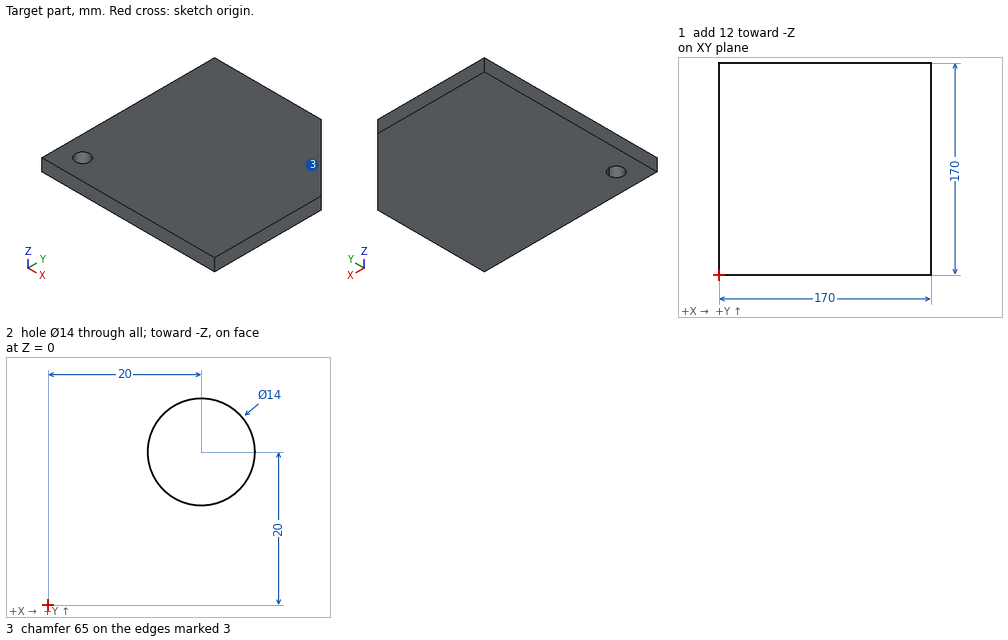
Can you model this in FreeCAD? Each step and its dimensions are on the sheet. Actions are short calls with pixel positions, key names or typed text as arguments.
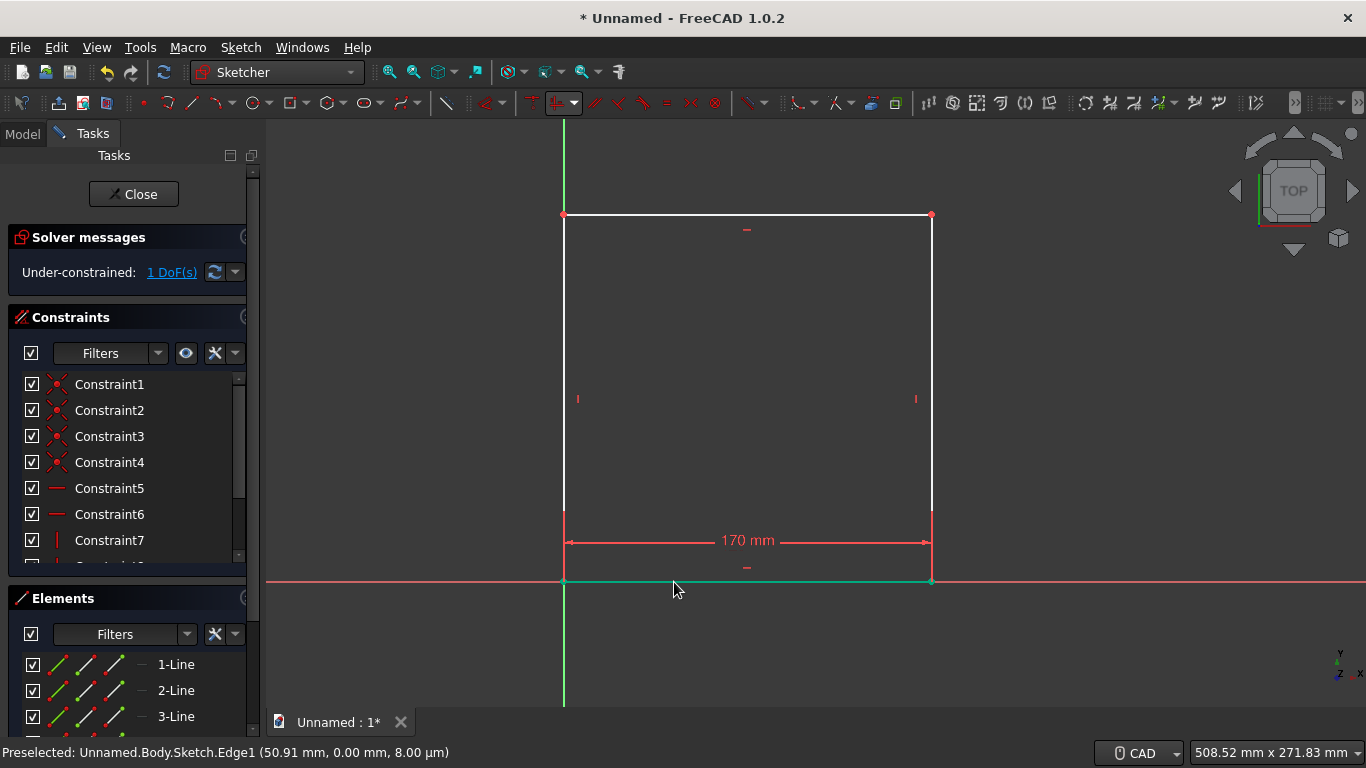
click(932, 472)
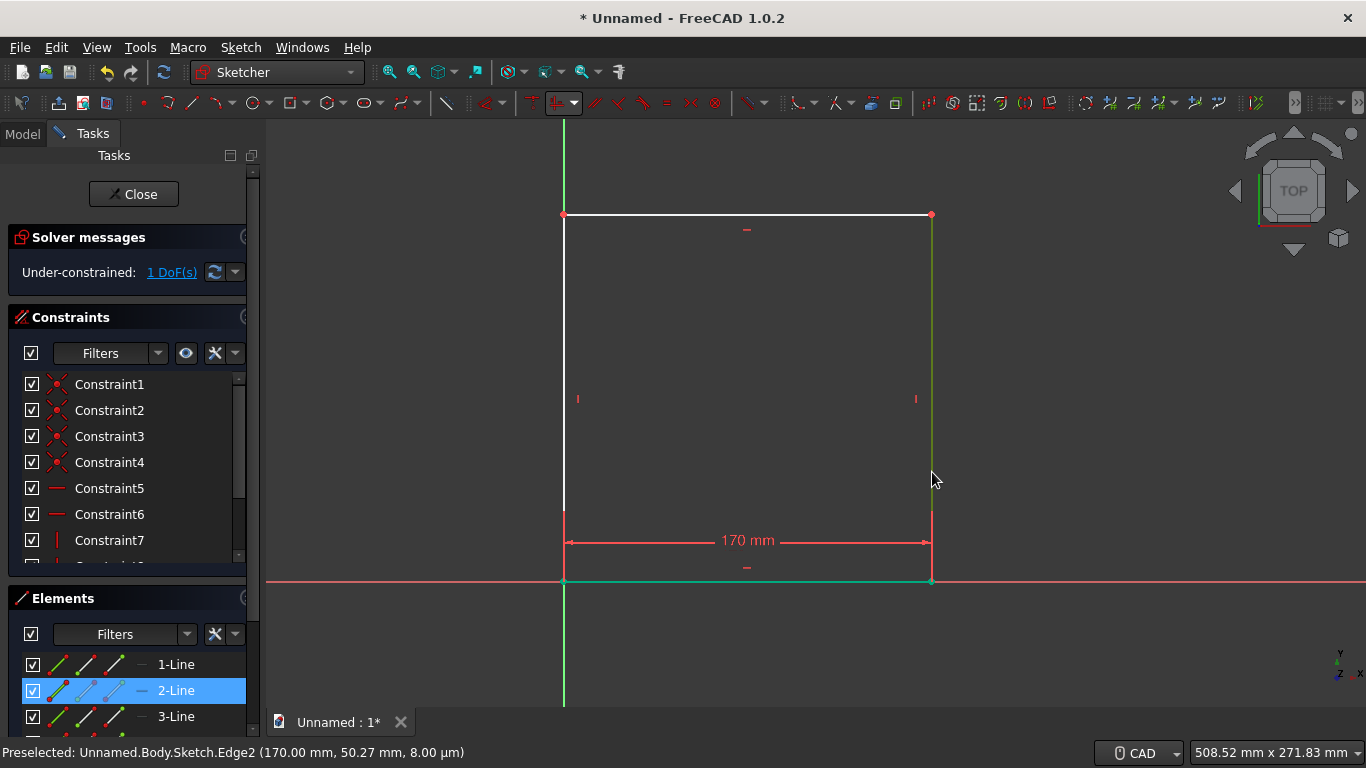
key(i)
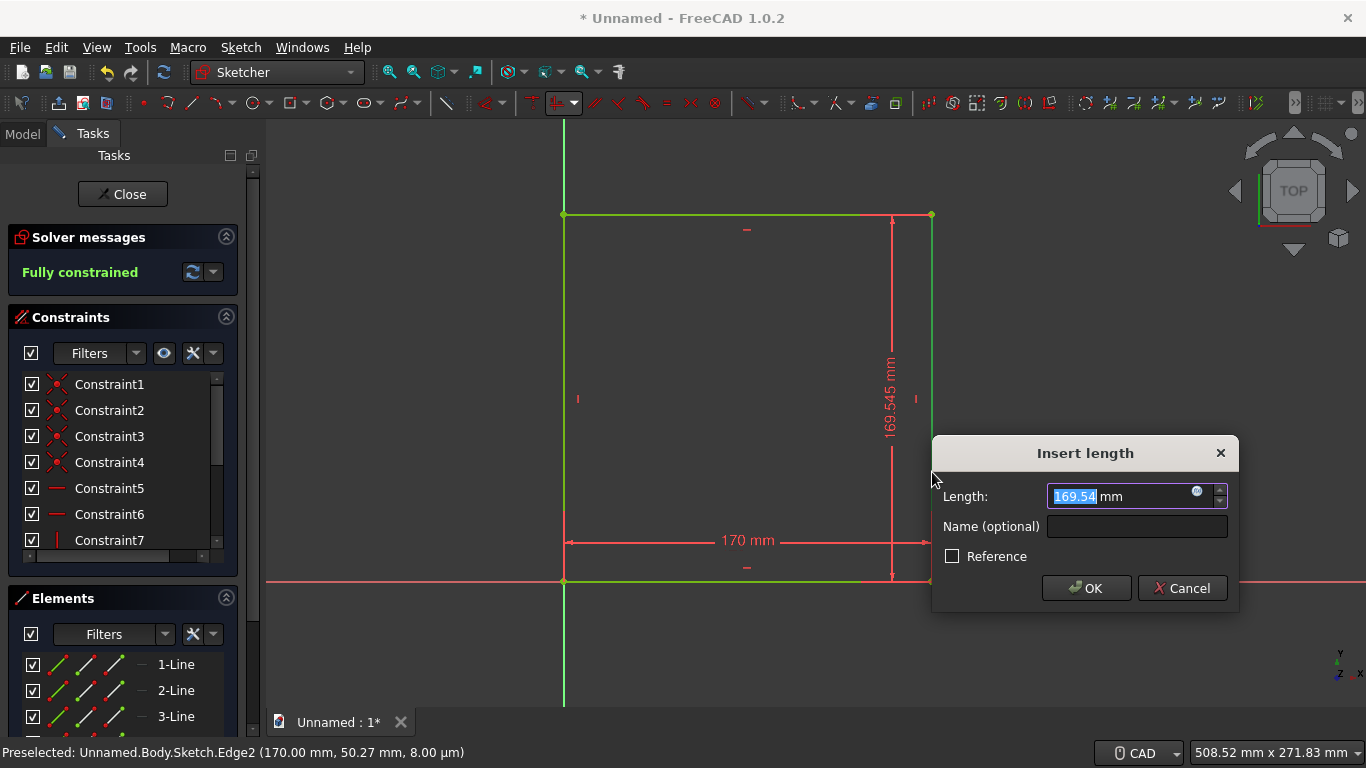
text(170)
key(Return)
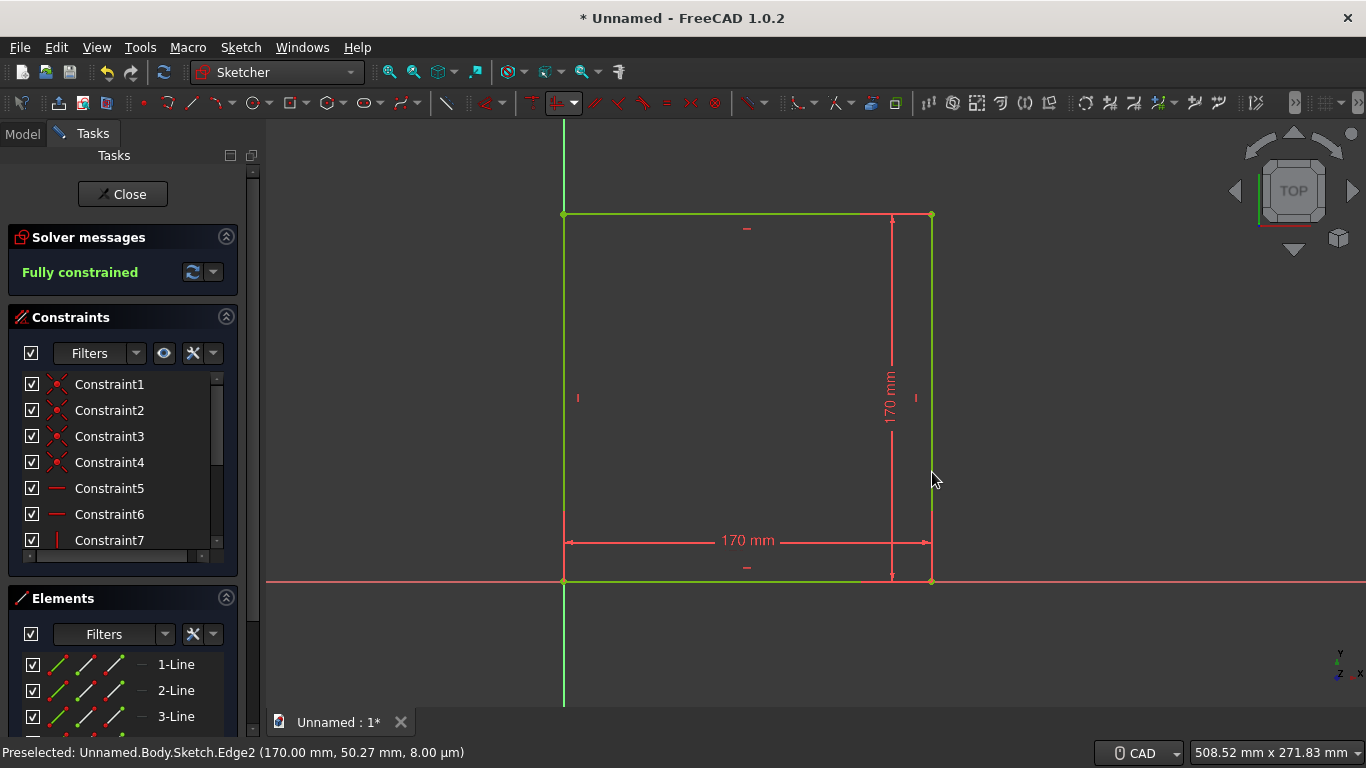
click(123, 194)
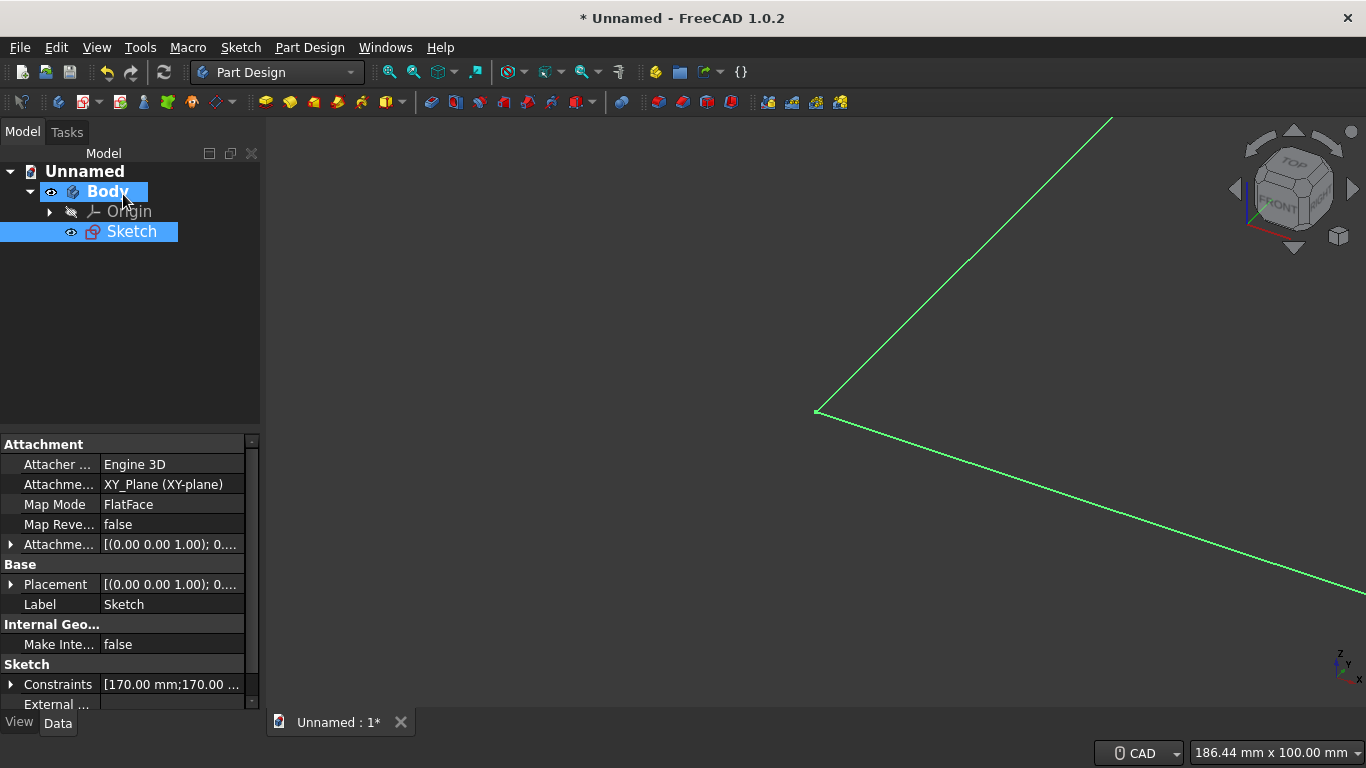
click(266, 102)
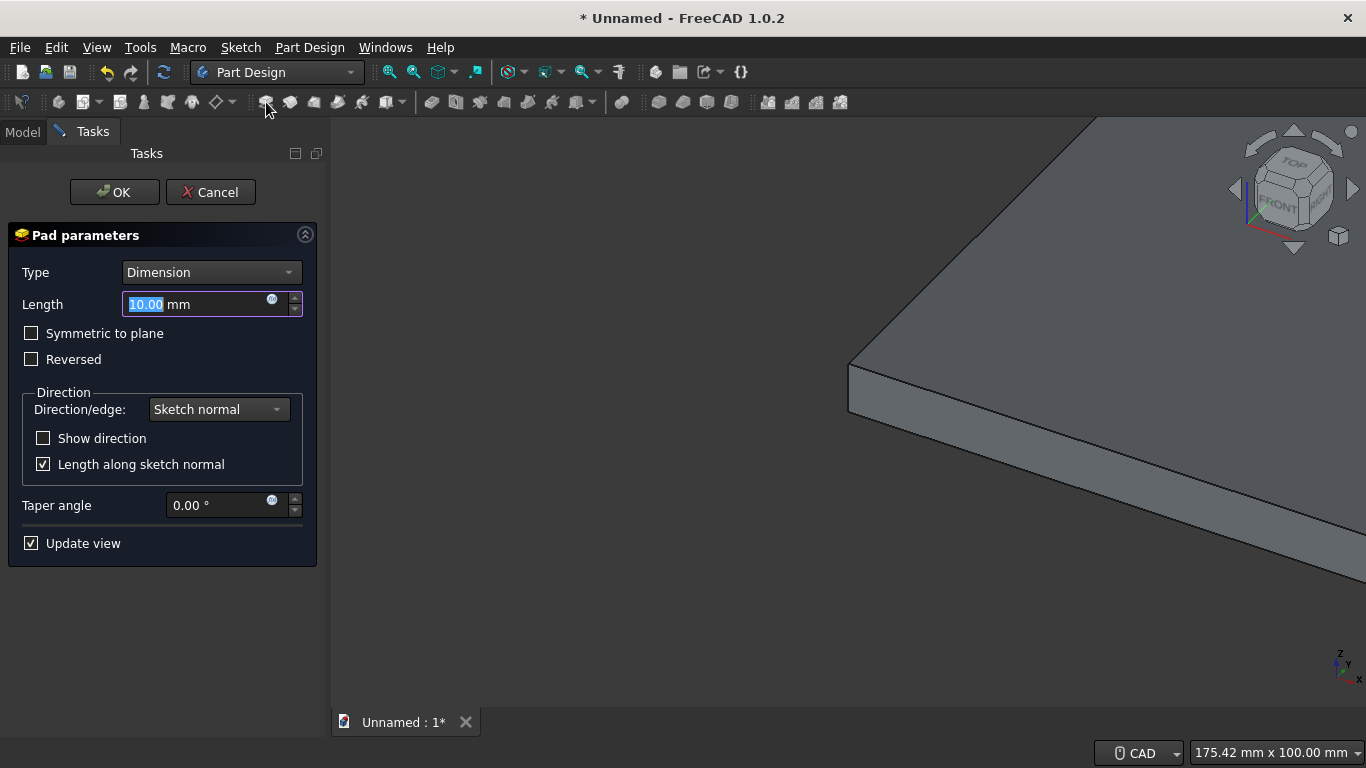
text(12)
key(Tab)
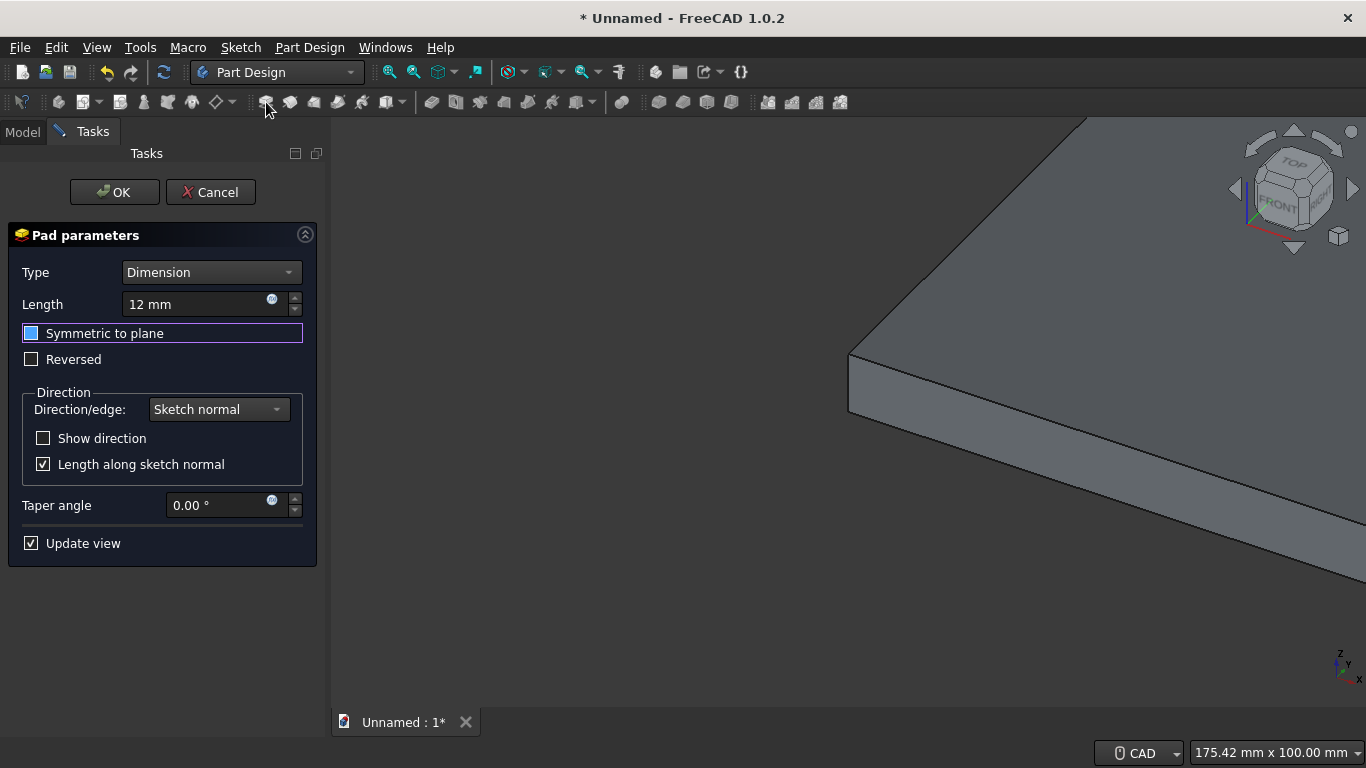
click(30, 359)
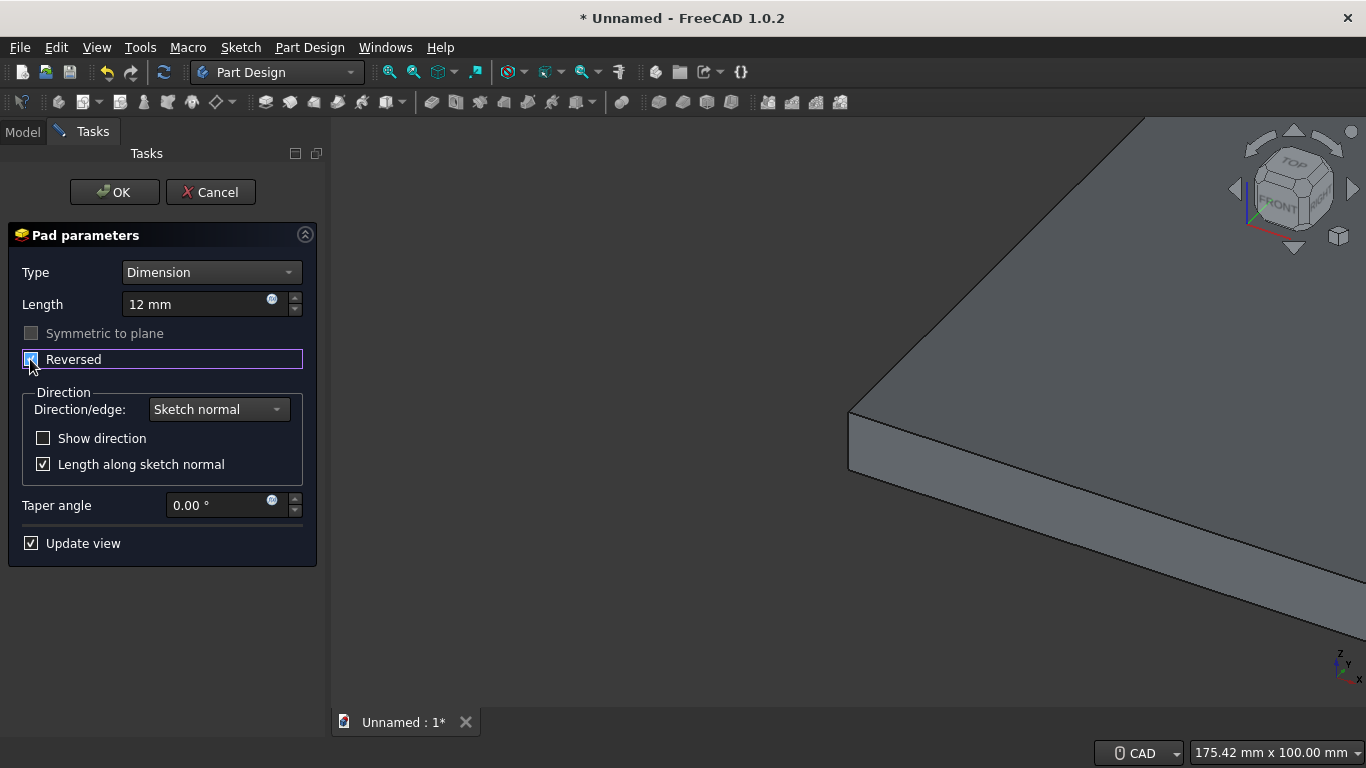
click(115, 192)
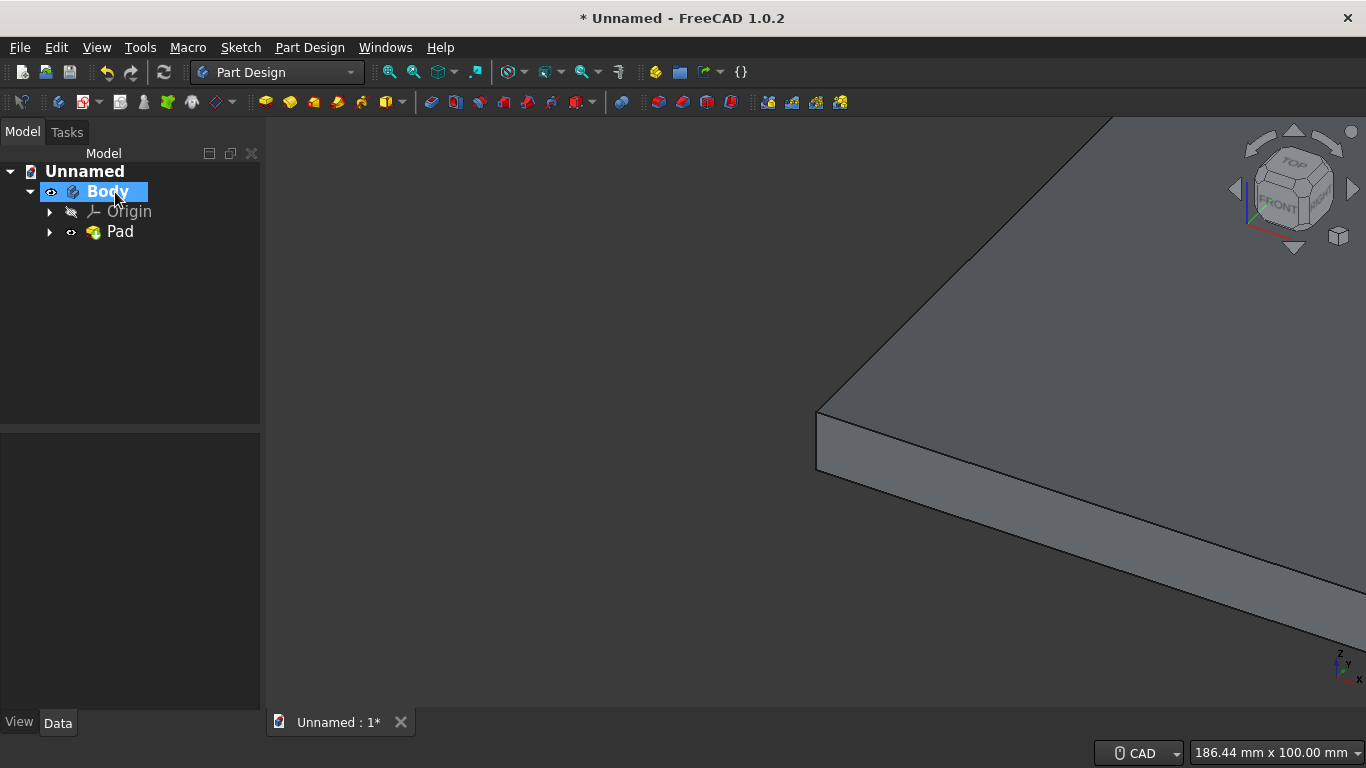
click(390, 72)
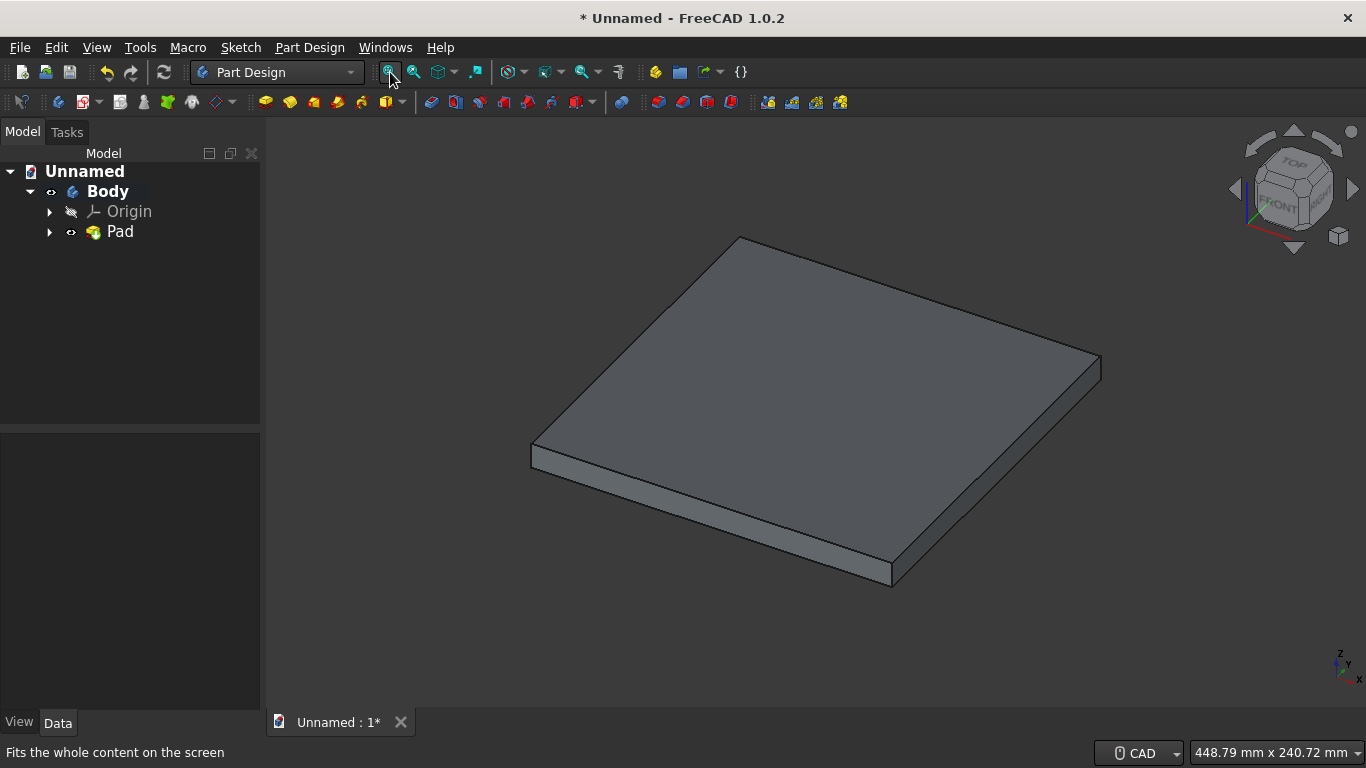
click(816, 399)